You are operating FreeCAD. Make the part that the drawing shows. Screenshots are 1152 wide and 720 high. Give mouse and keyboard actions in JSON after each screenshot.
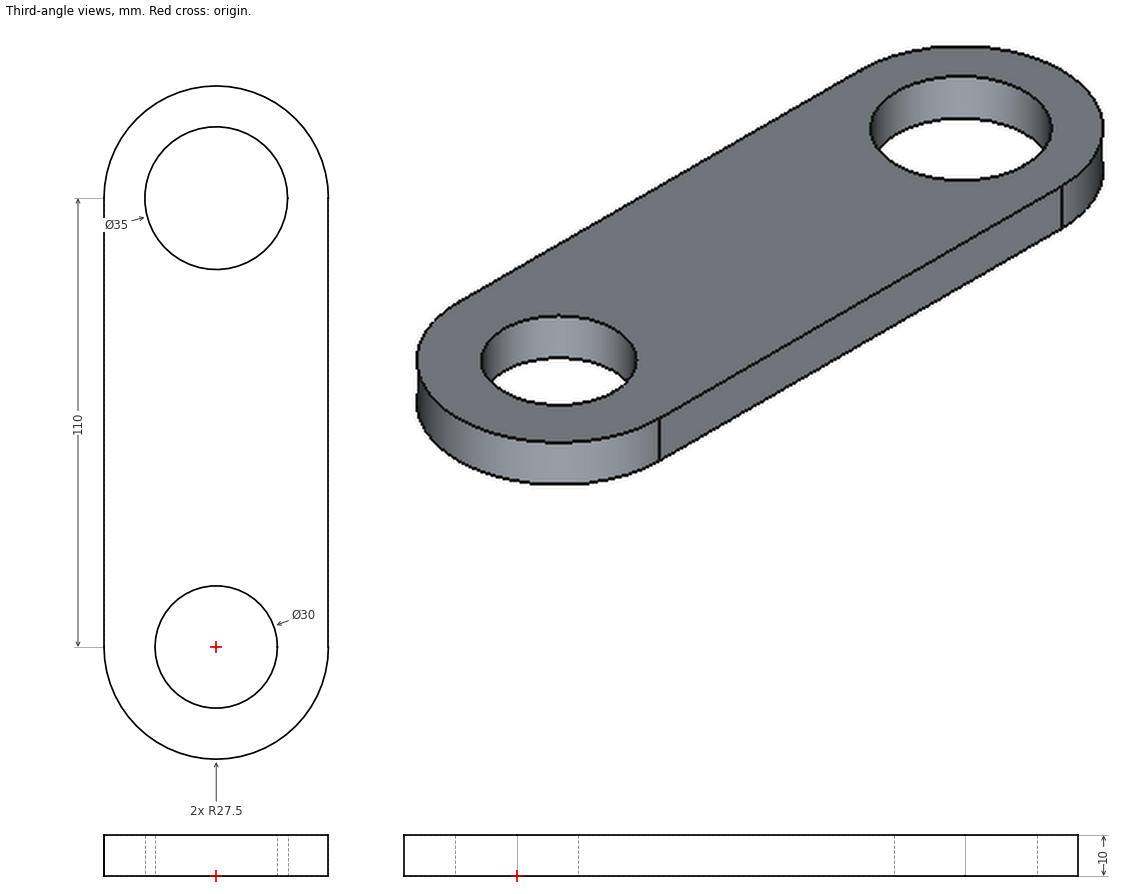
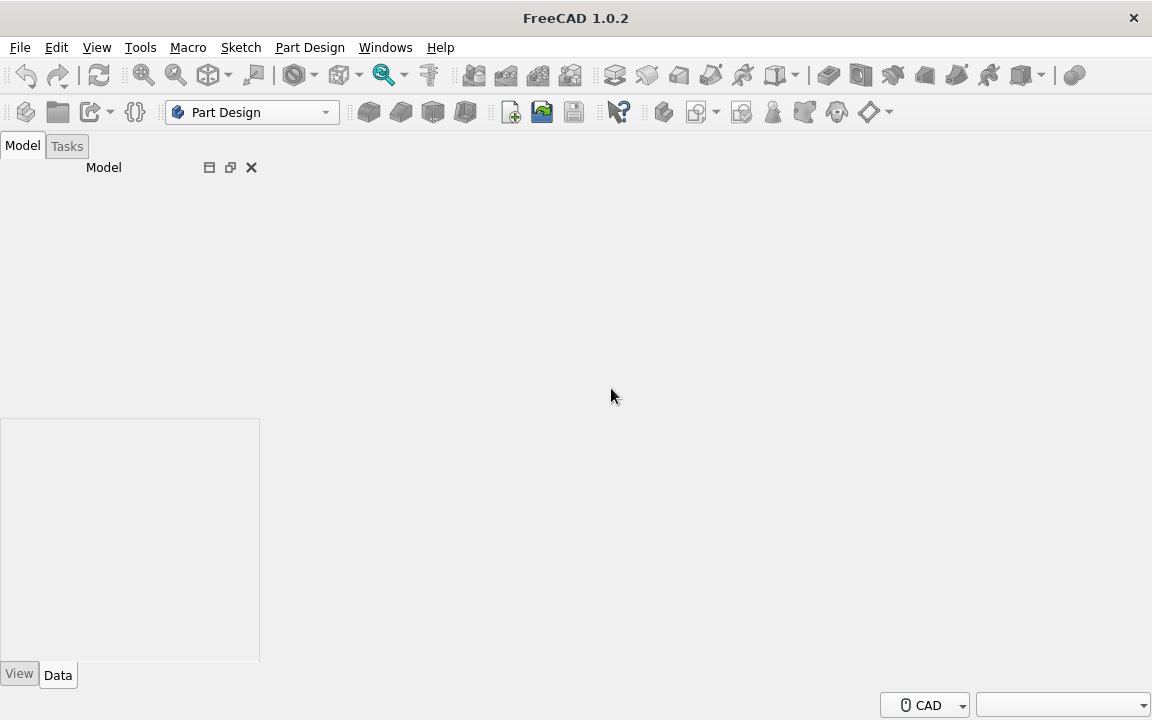
{"action": "left_click", "coordinate": [510, 112]}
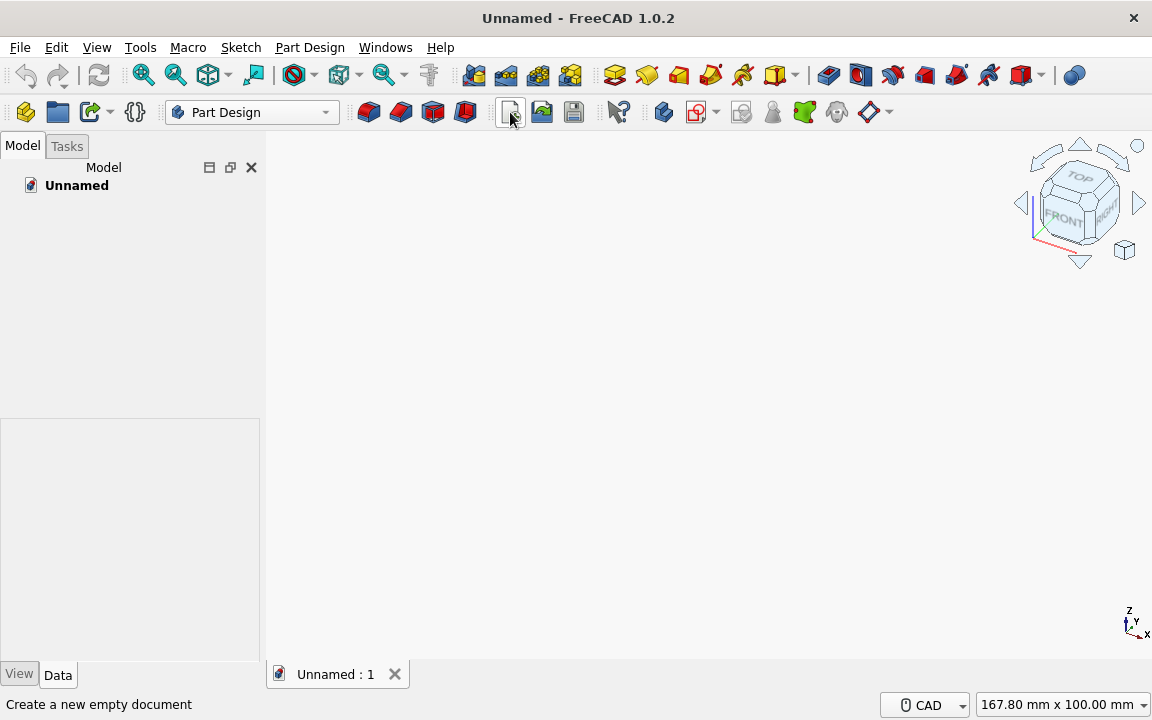
{"action": "left_click", "coordinate": [696, 112]}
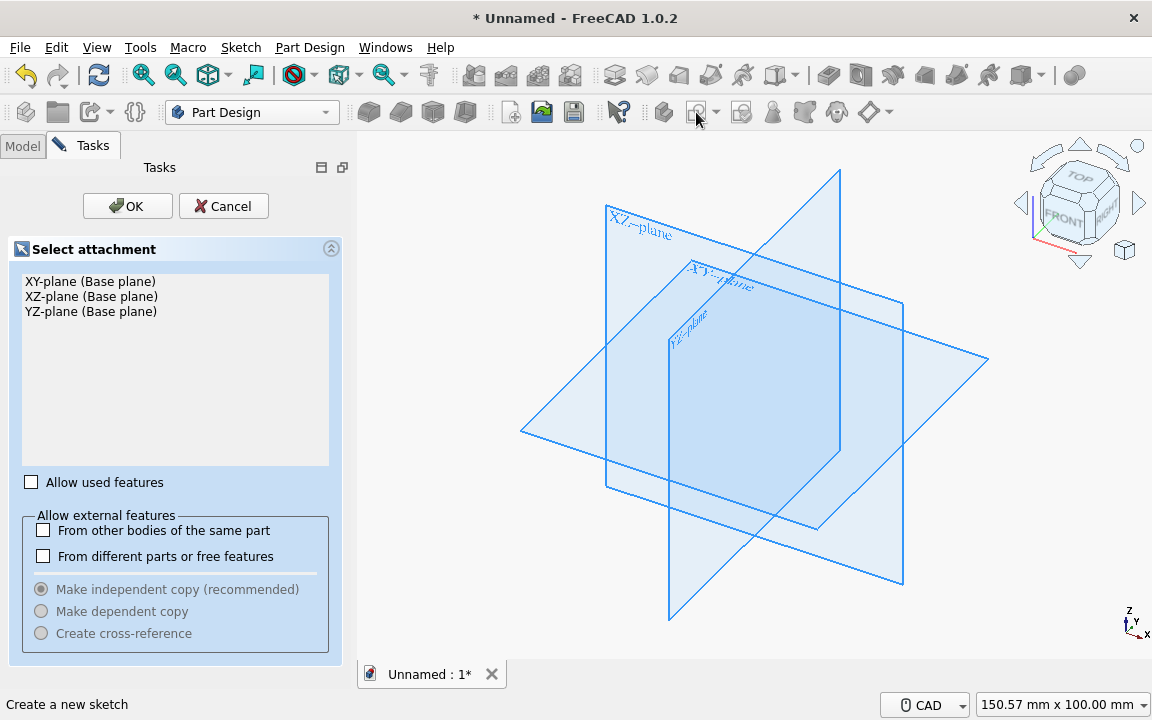
{"action": "left_click", "coordinate": [82, 282]}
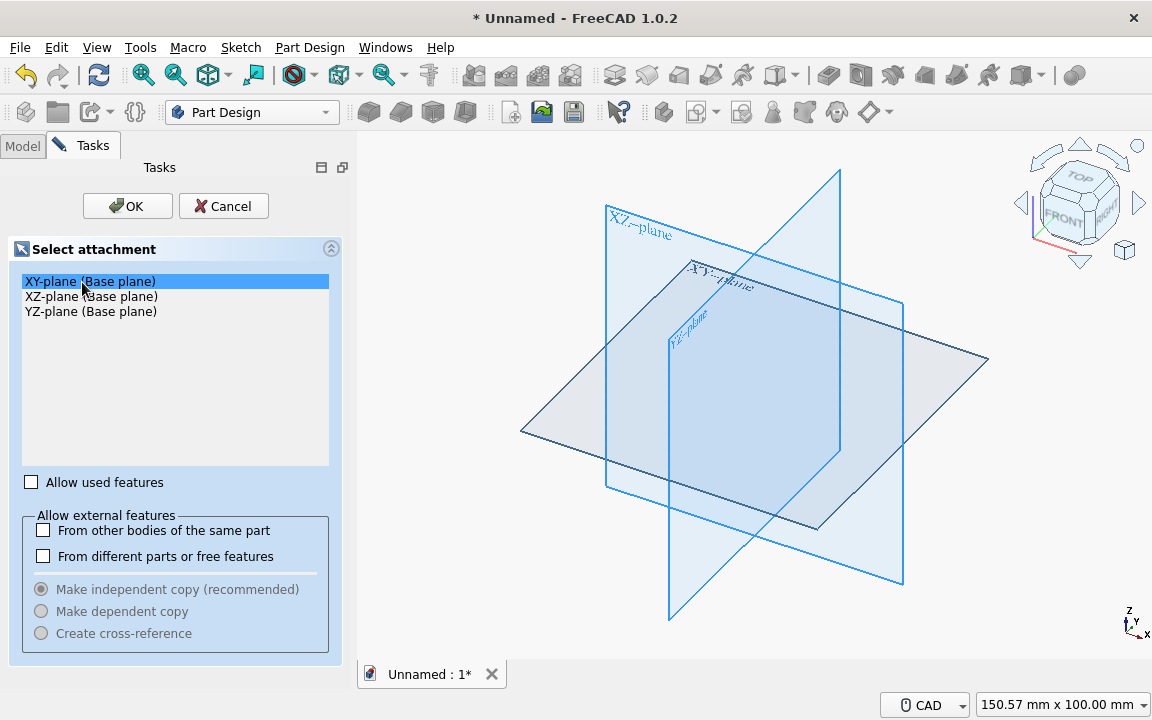
{"action": "left_click", "coordinate": [128, 206]}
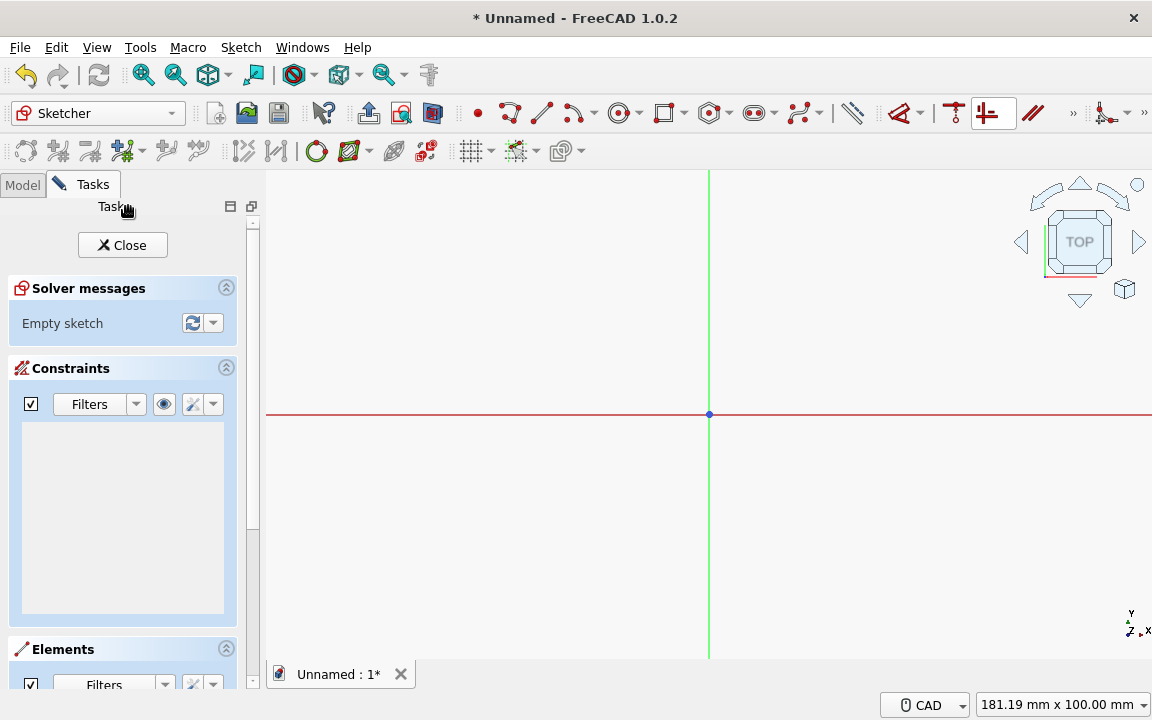
{"action": "scroll", "coordinate": [601, 571], "scroll_direction": "down", "scroll_amount": 5}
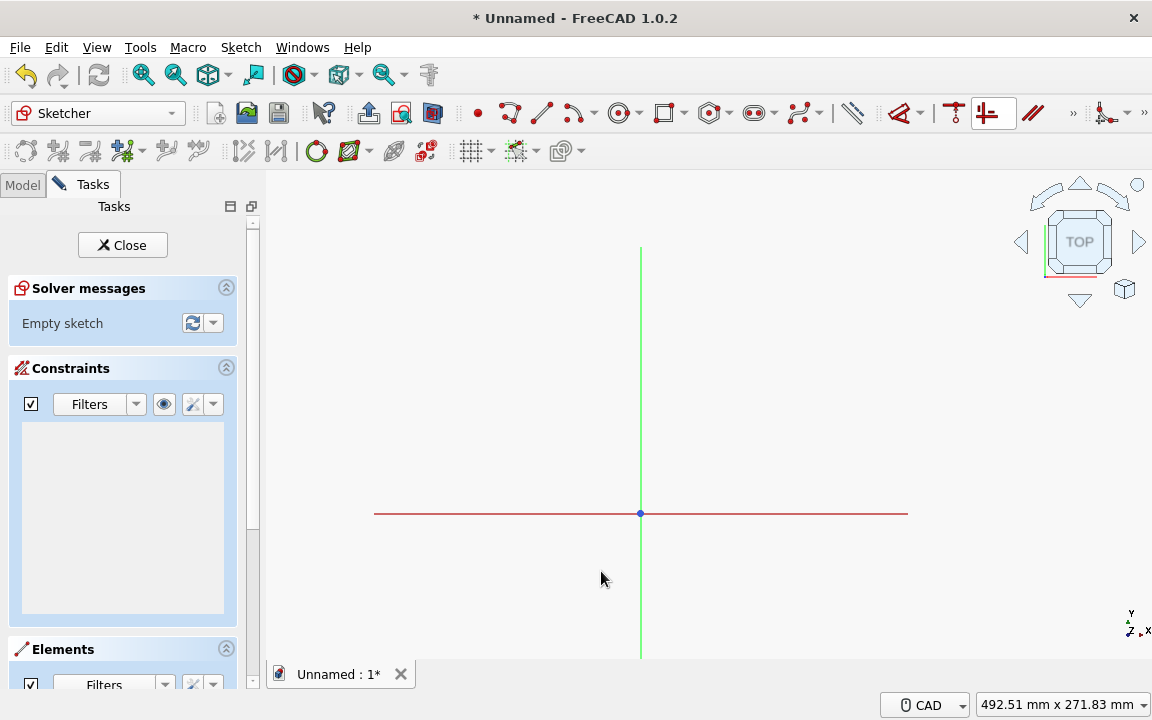
{"action": "key", "text": "g s"}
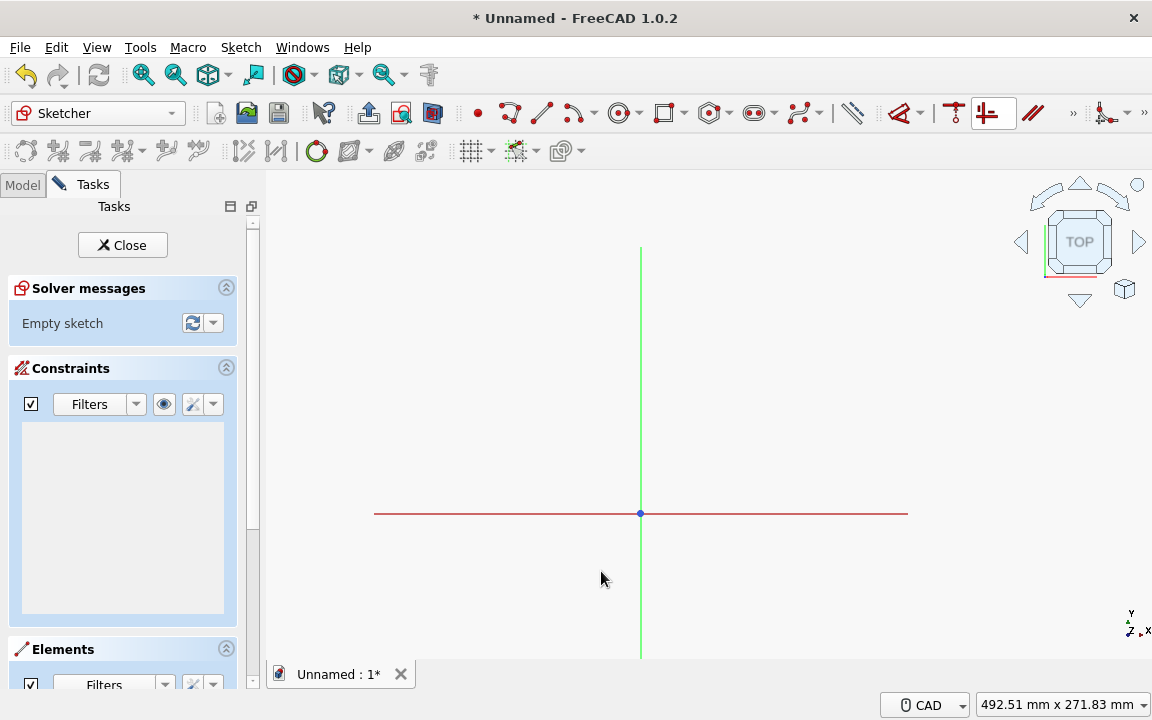
{"action": "left_click", "coordinate": [641, 514]}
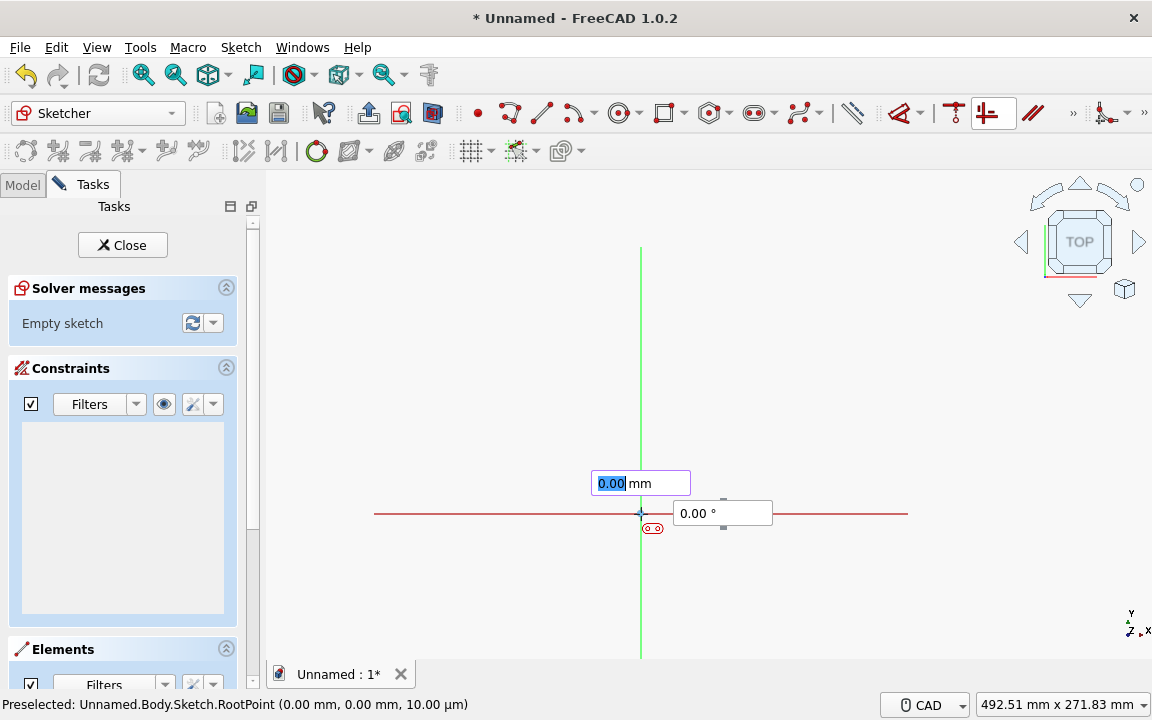
{"action": "left_click", "coordinate": [650, 316]}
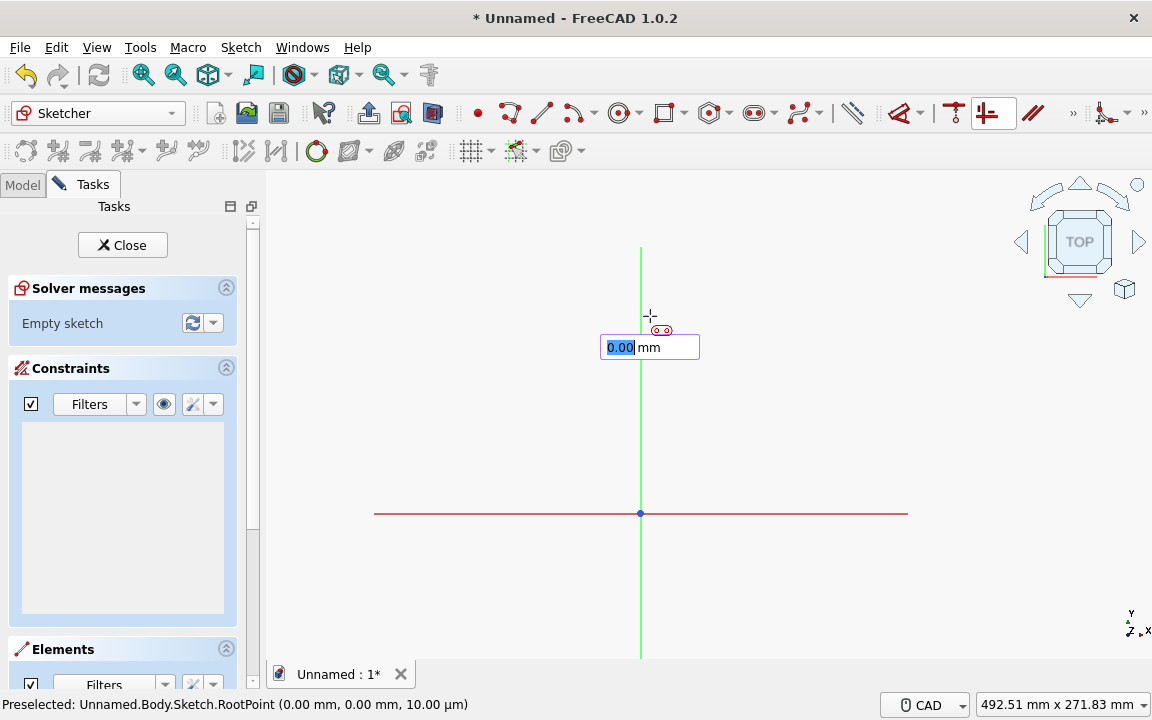
{"action": "left_click", "coordinate": [591, 415]}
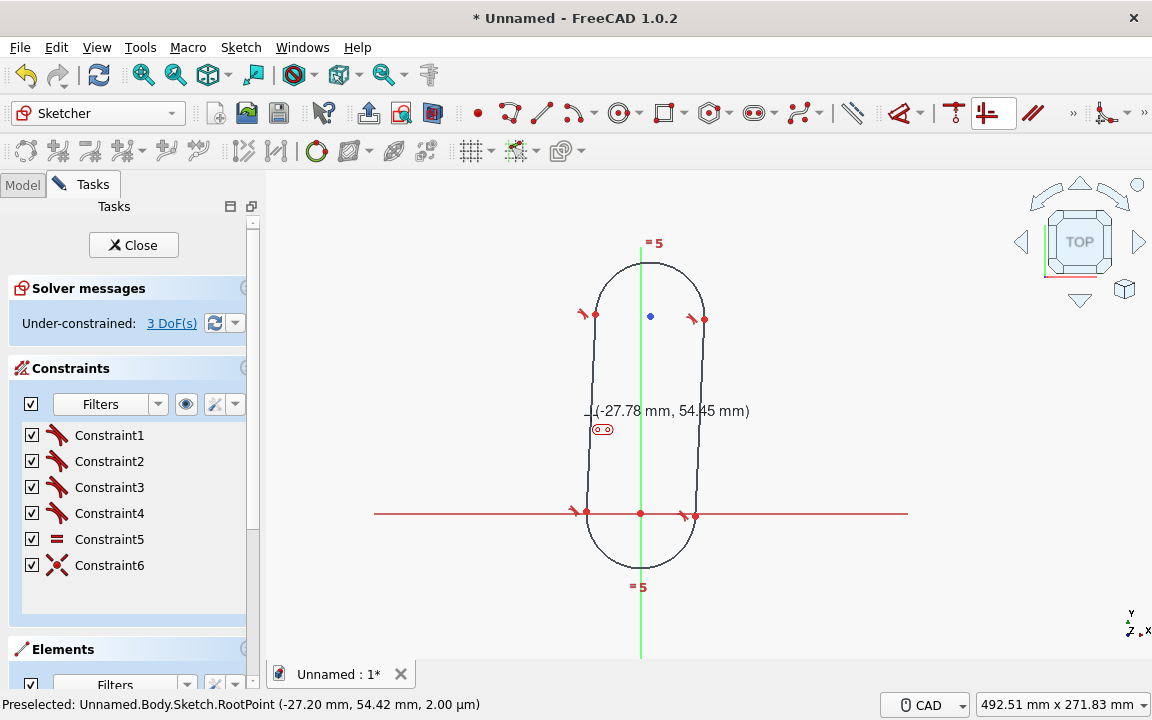
{"action": "left_click", "coordinate": [620, 114]}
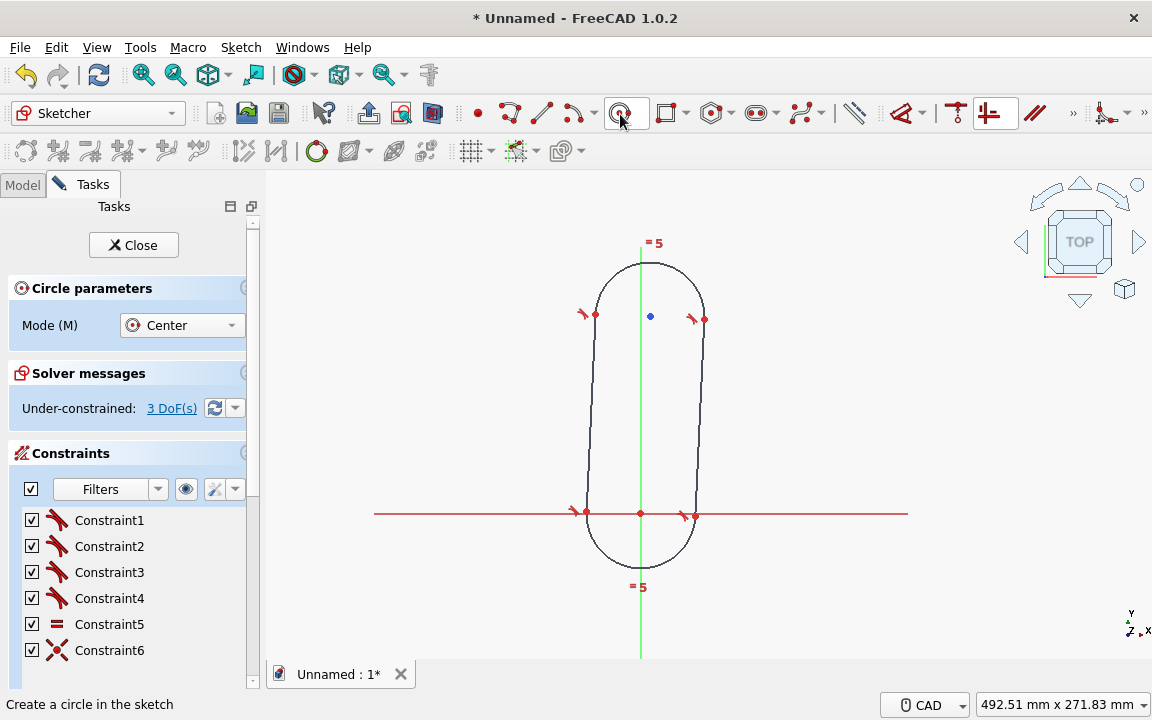
{"action": "left_click", "coordinate": [641, 514]}
{"action": "left_click", "coordinate": [660, 495]}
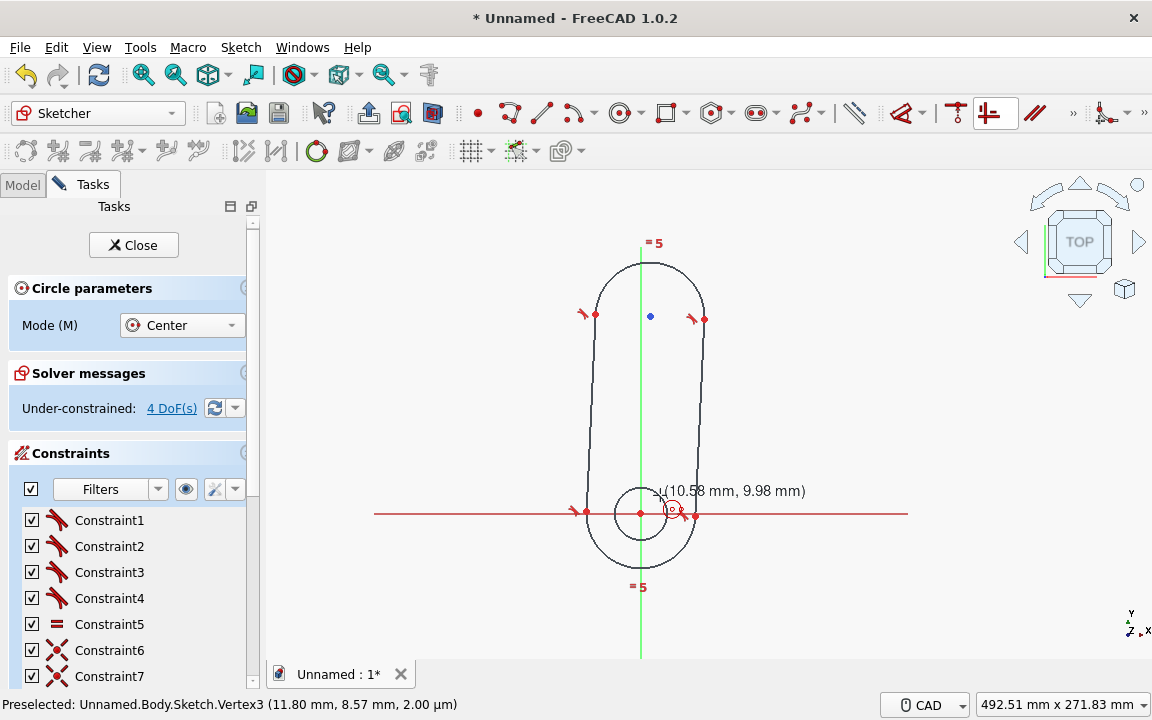
{"action": "left_click", "coordinate": [650, 317]}
{"action": "left_click", "coordinate": [663, 294]}
{"action": "key", "text": "Escape"}